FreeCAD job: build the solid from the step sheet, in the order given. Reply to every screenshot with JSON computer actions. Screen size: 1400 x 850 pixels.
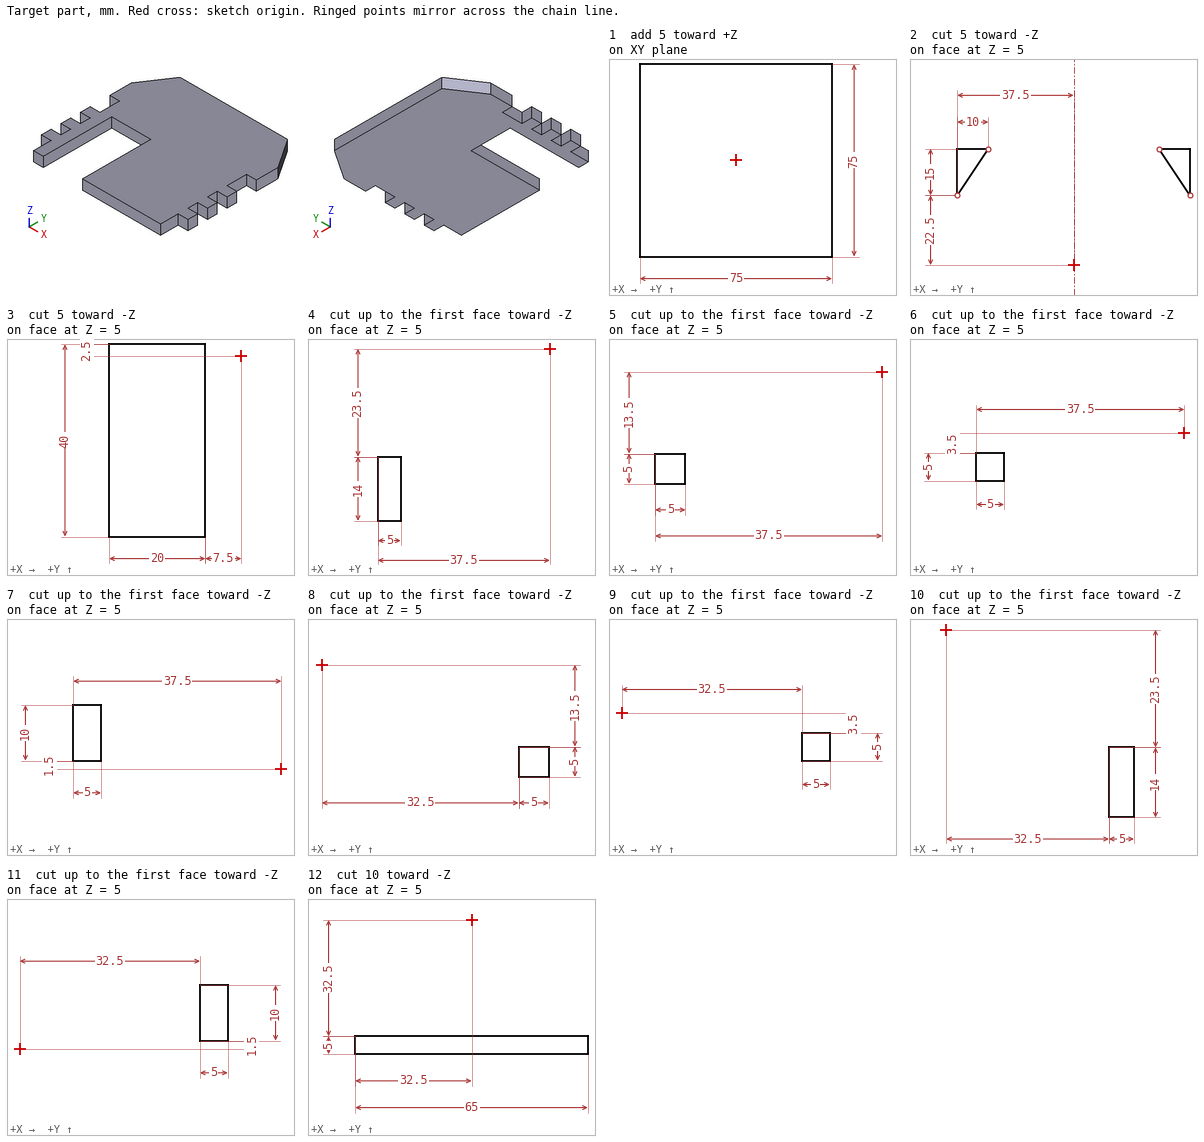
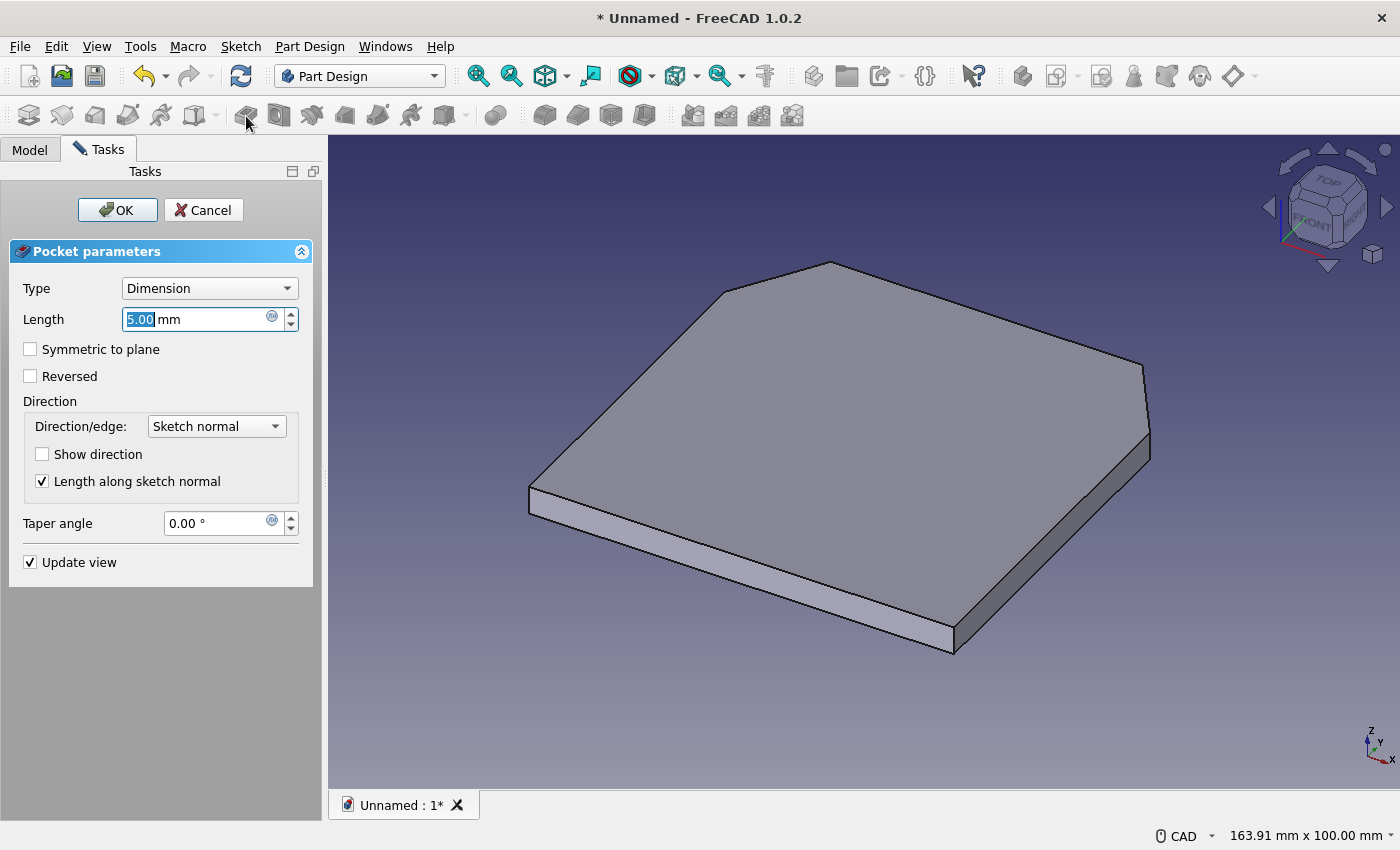
{"action": "type", "text": "5"}
{"action": "key", "text": "Tab"}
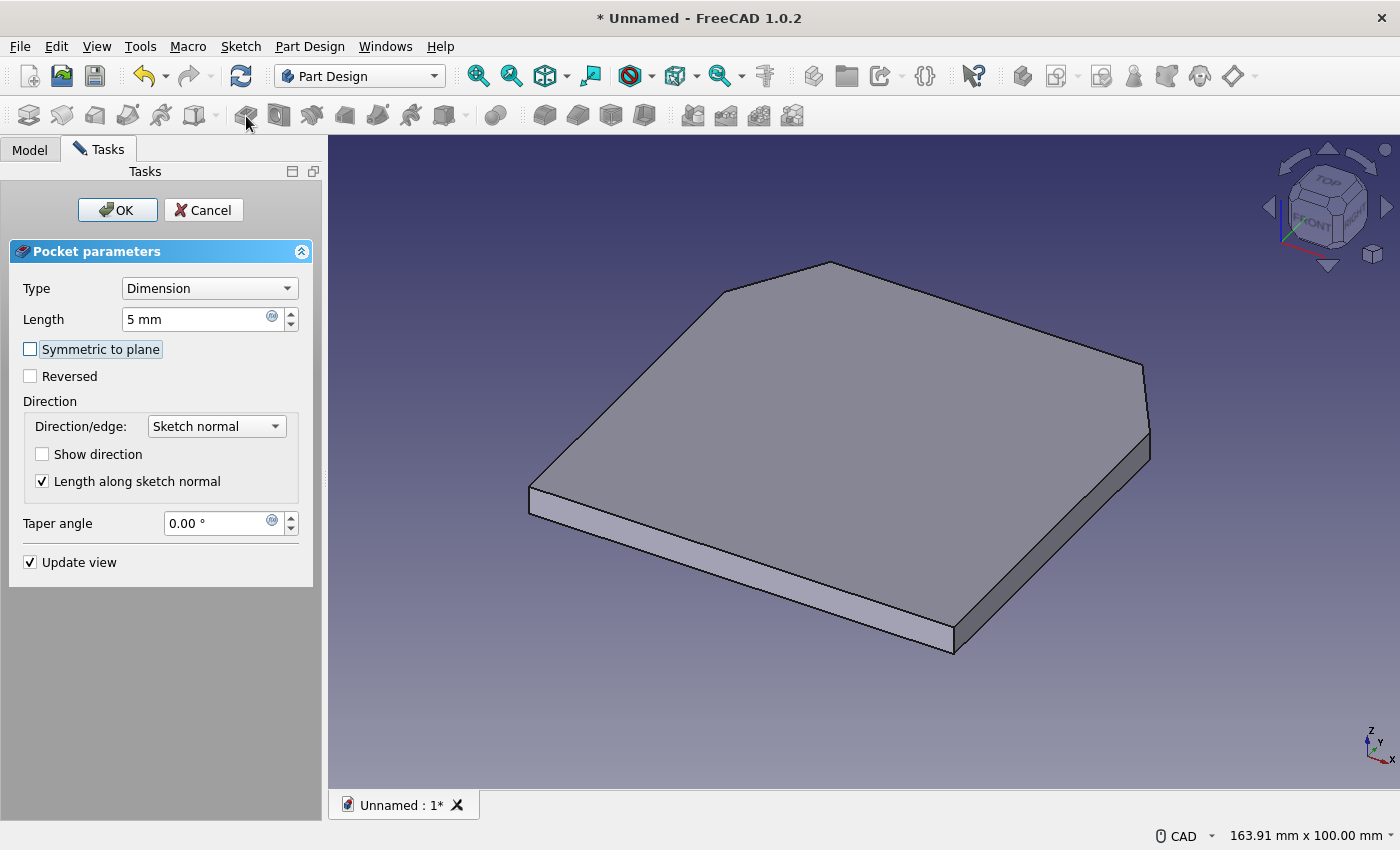
{"action": "left_click", "coordinate": [118, 210]}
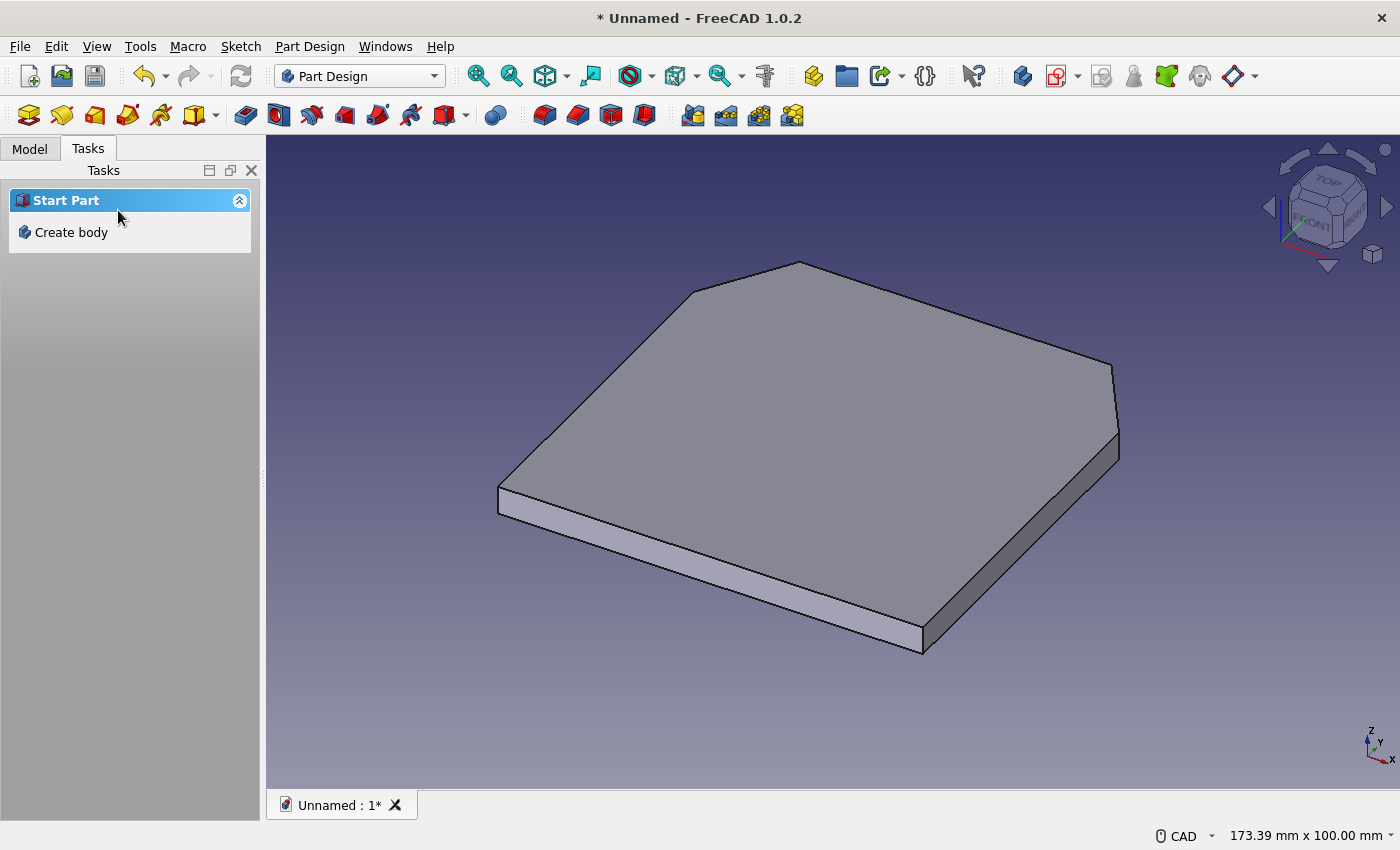
{"action": "left_click", "coordinate": [833, 434]}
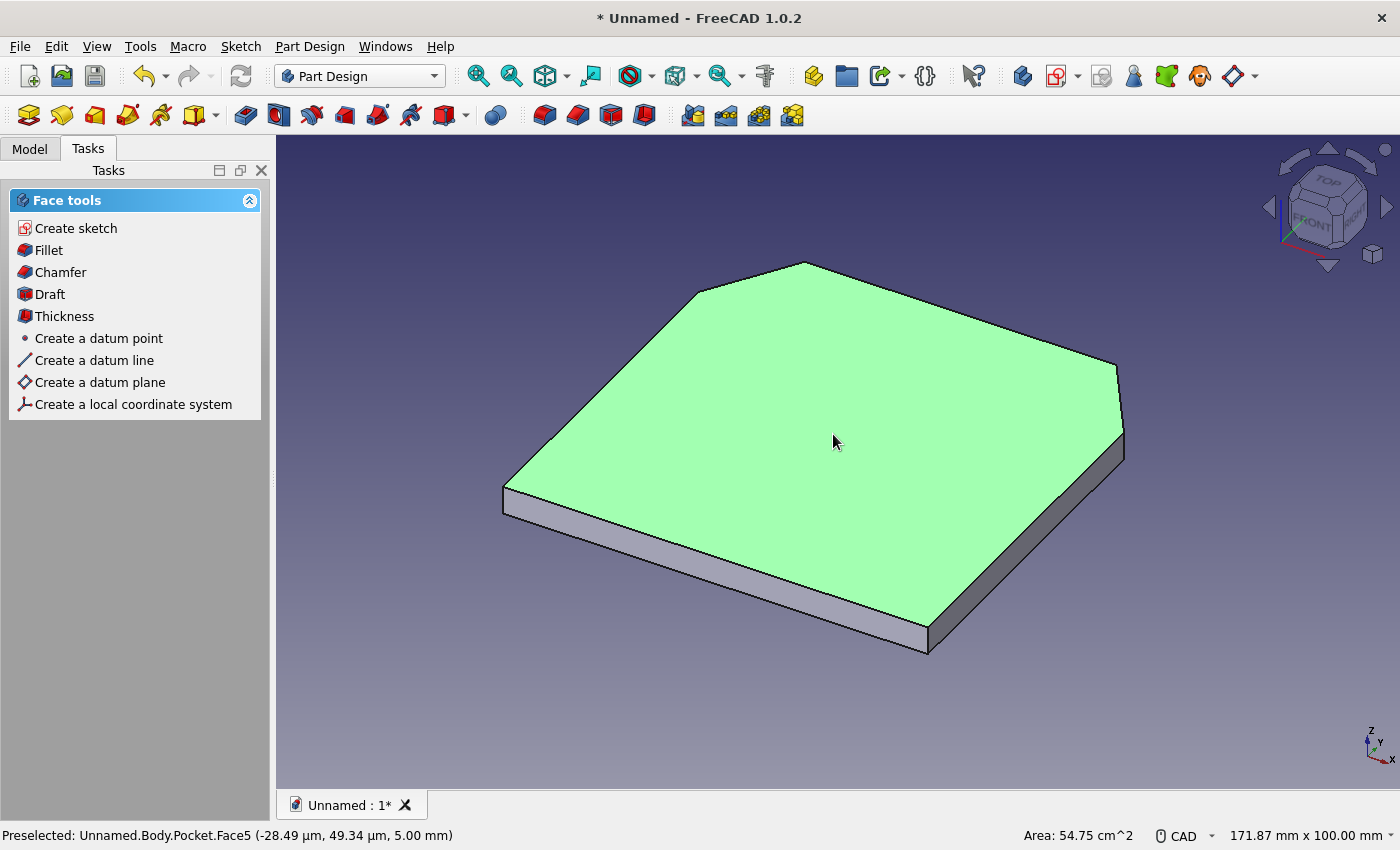
{"action": "left_click", "coordinate": [1056, 76]}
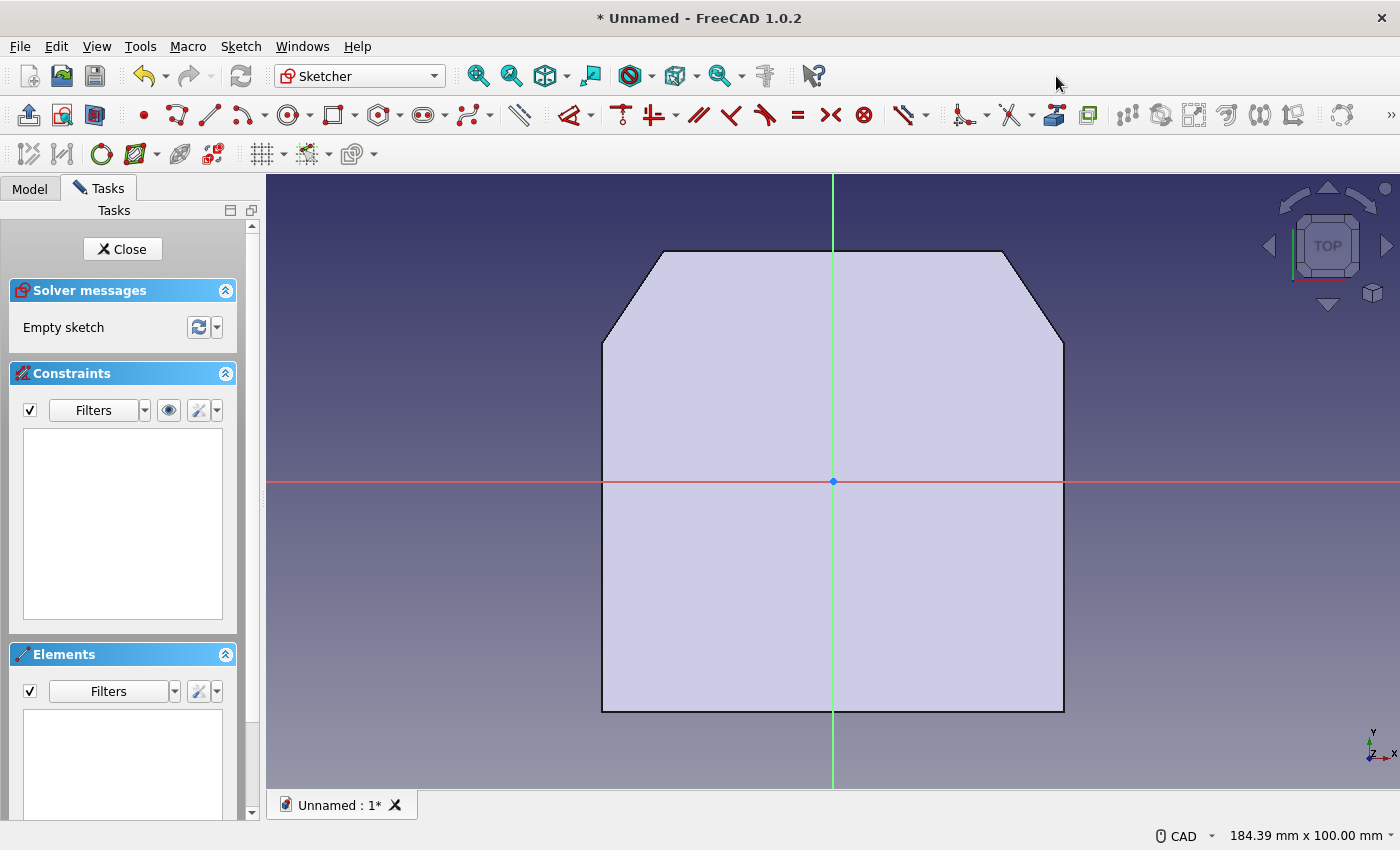
{"action": "scroll", "coordinate": [716, 761], "scroll_direction": "up", "scroll_amount": 2}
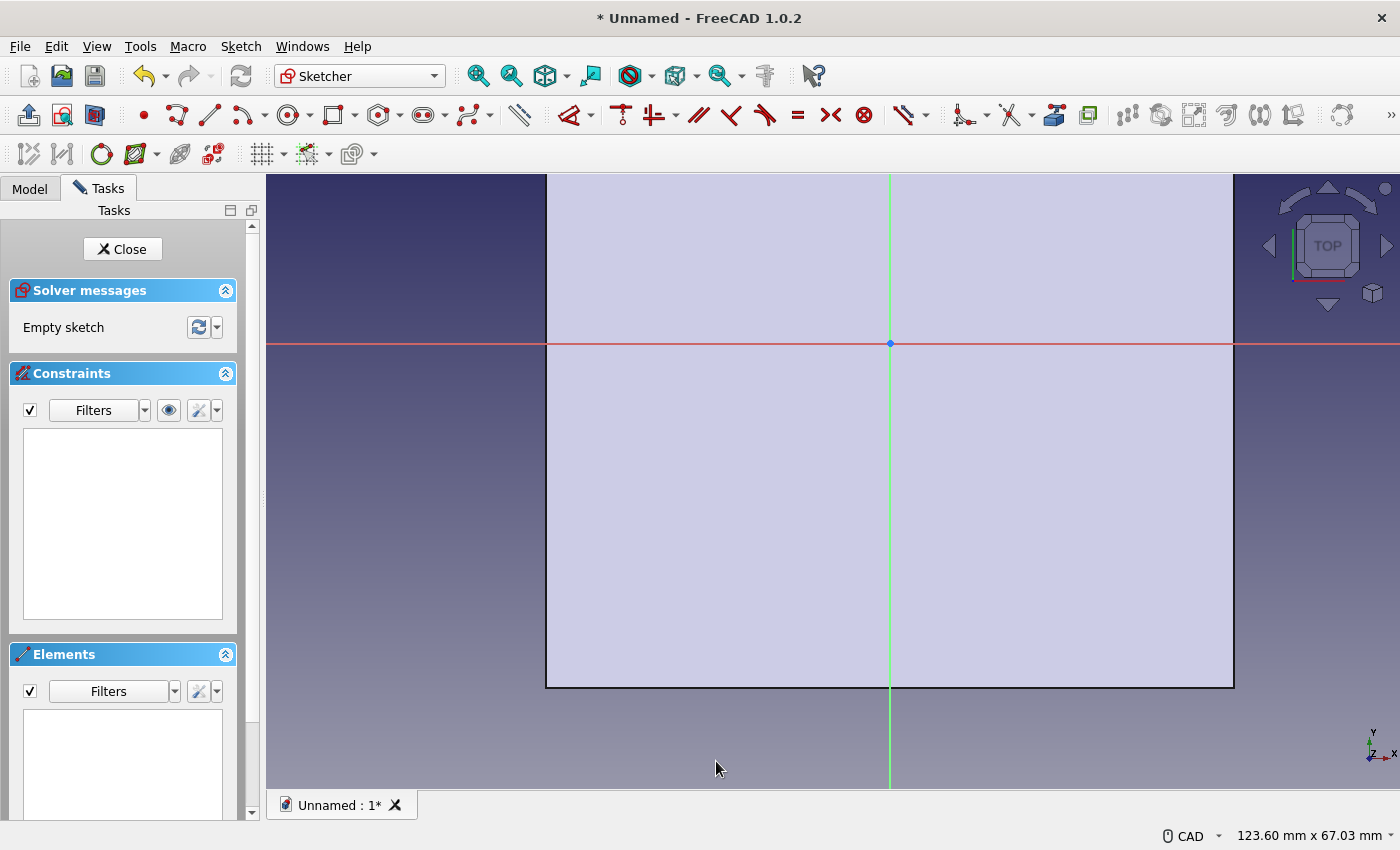
{"action": "key", "text": "g r"}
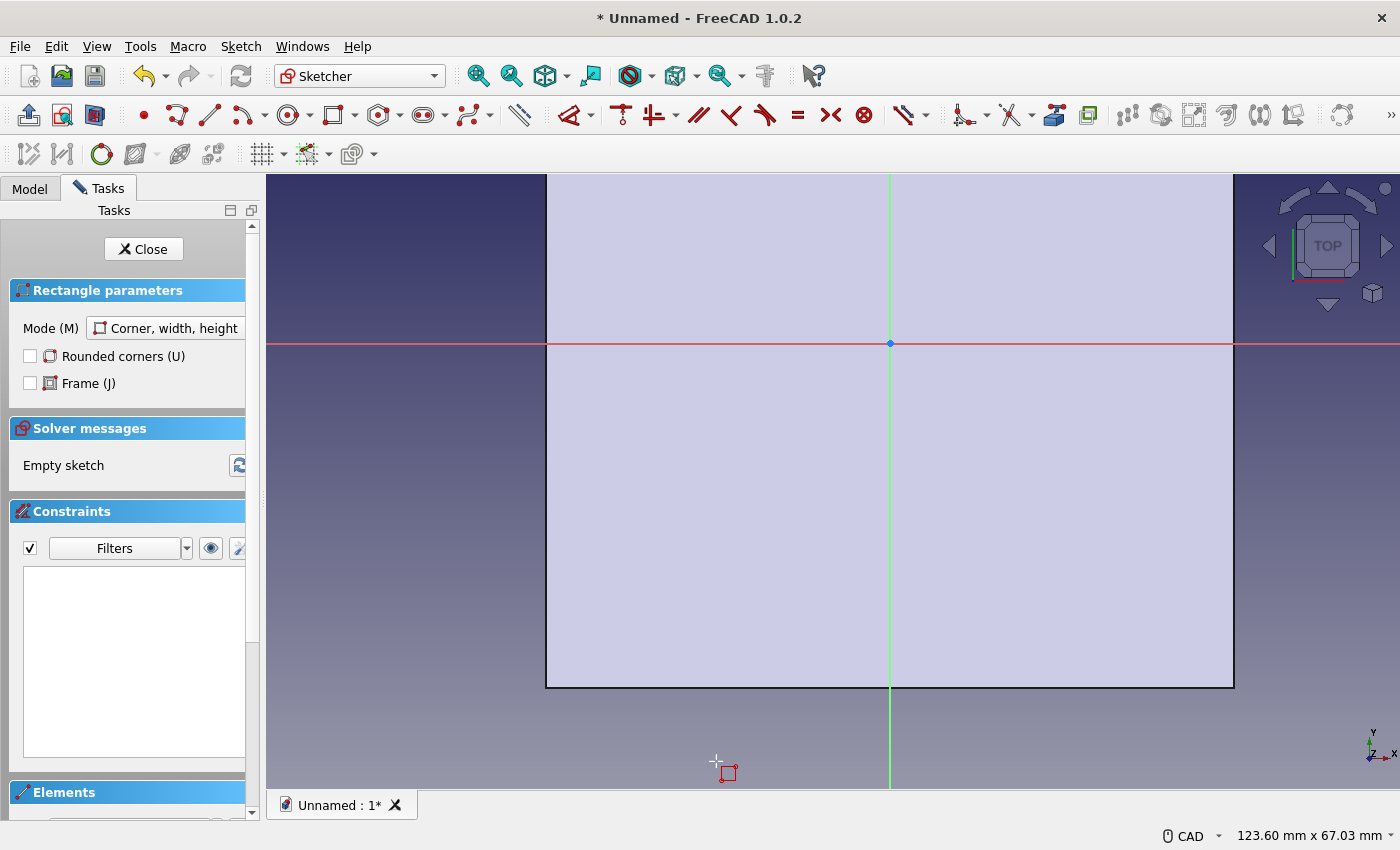
{"action": "left_click", "coordinate": [638, 321]}
{"action": "left_click", "coordinate": [822, 688]}
{"action": "key", "text": "Escape"}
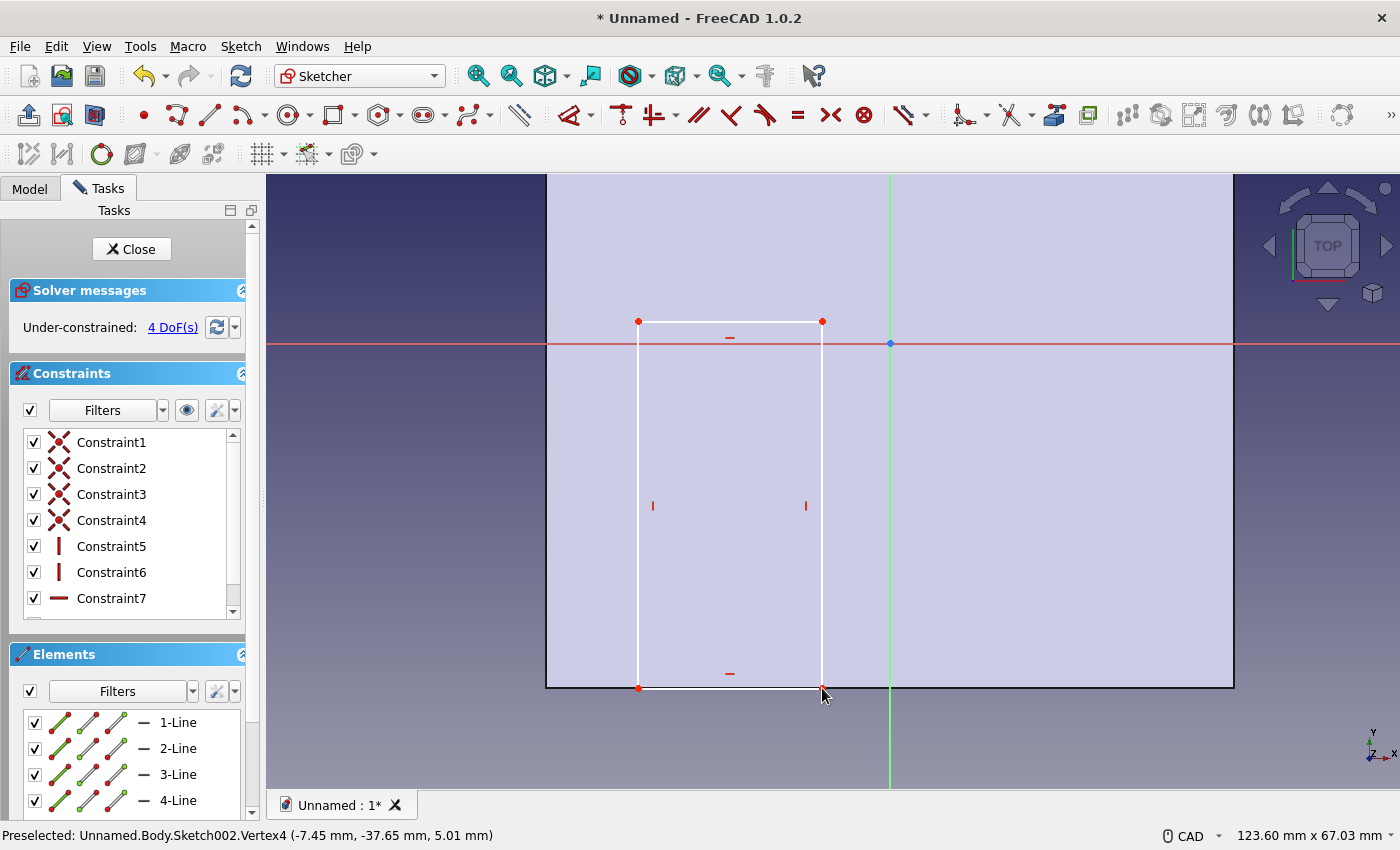
{"action": "left_click", "coordinate": [568, 116]}